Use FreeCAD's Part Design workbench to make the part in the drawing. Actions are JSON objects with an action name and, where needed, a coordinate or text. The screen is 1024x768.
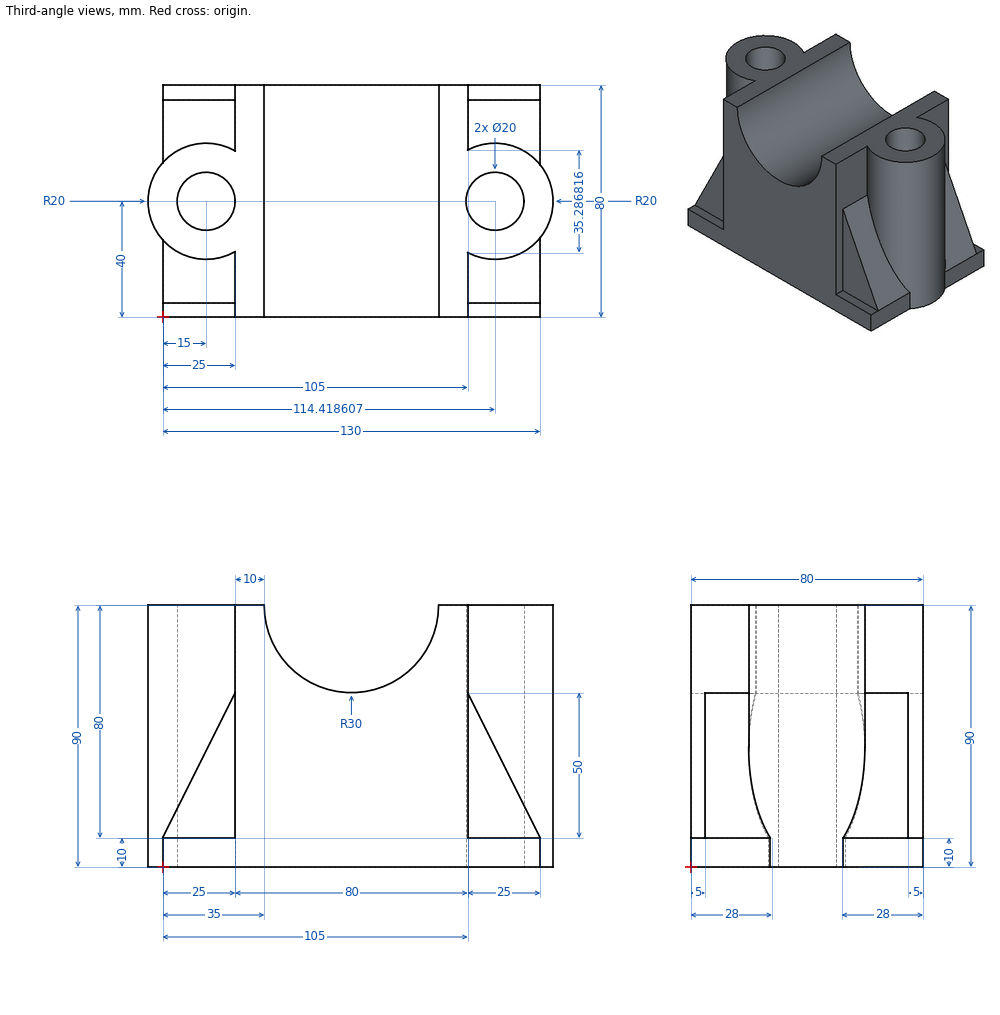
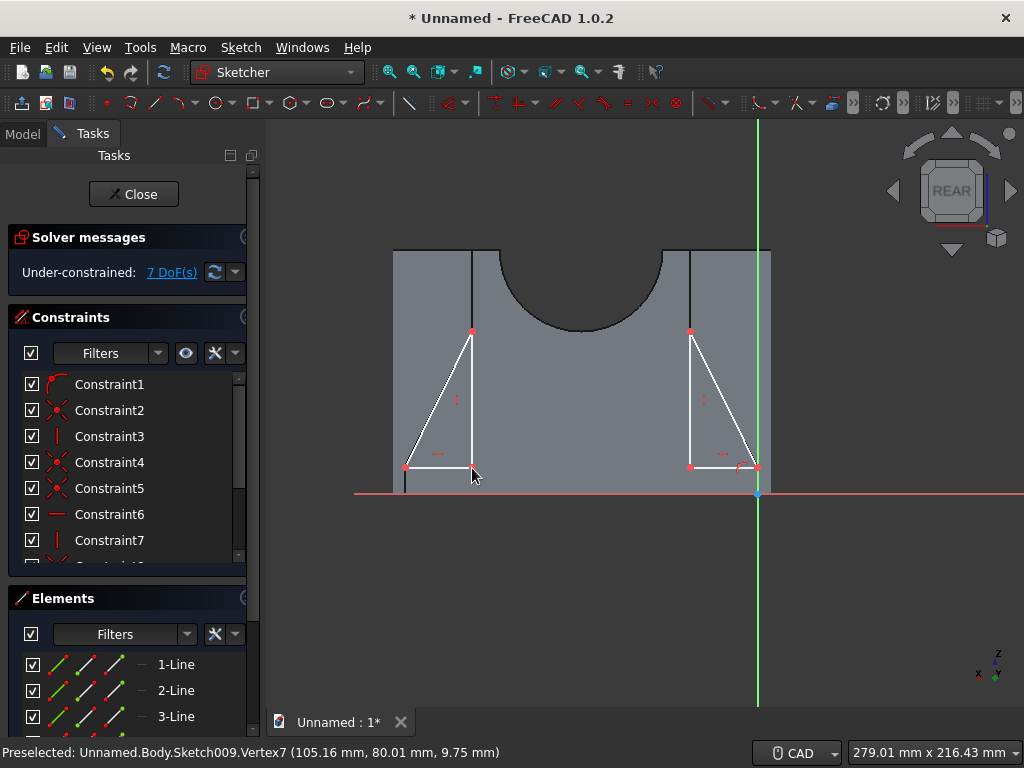
{"action": "left_click", "coordinate": [448, 104]}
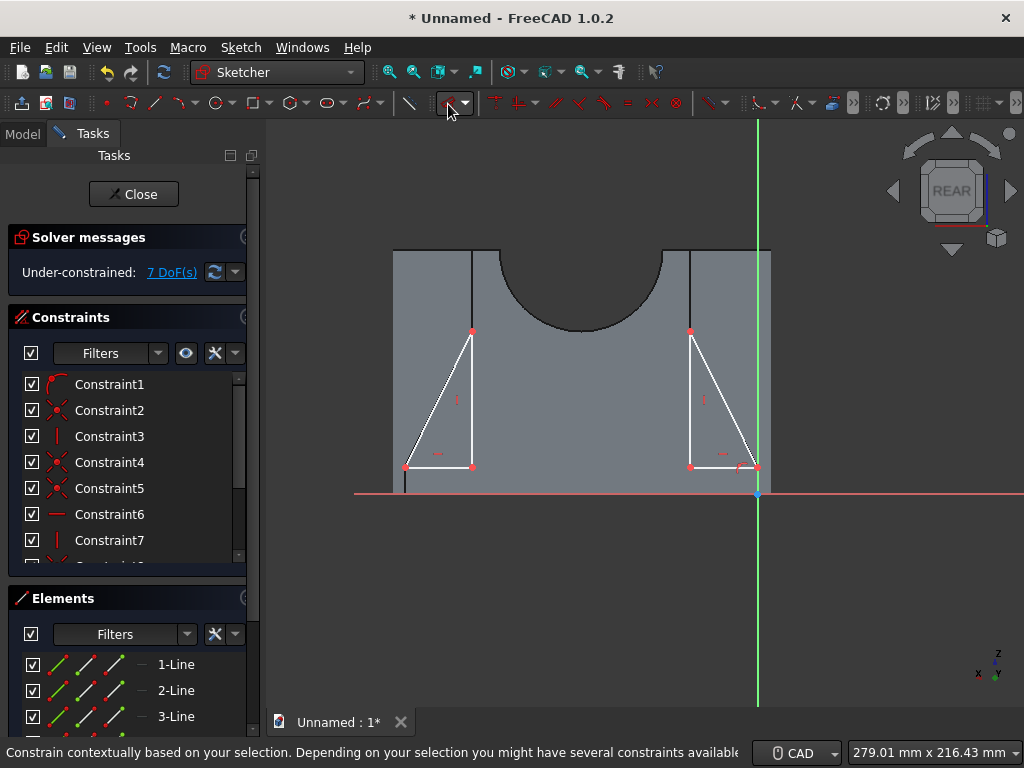
{"action": "left_click", "coordinate": [690, 373]}
{"action": "left_click", "coordinate": [724, 369]}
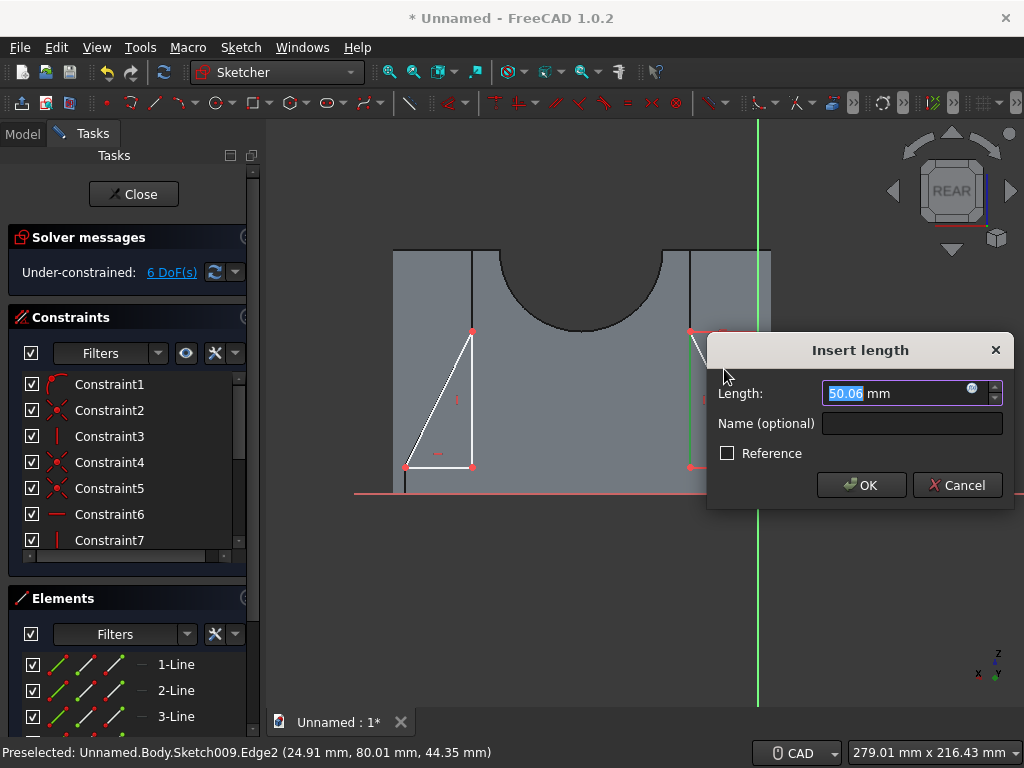
{"action": "type", "text": "50"}
{"action": "key", "text": "Return"}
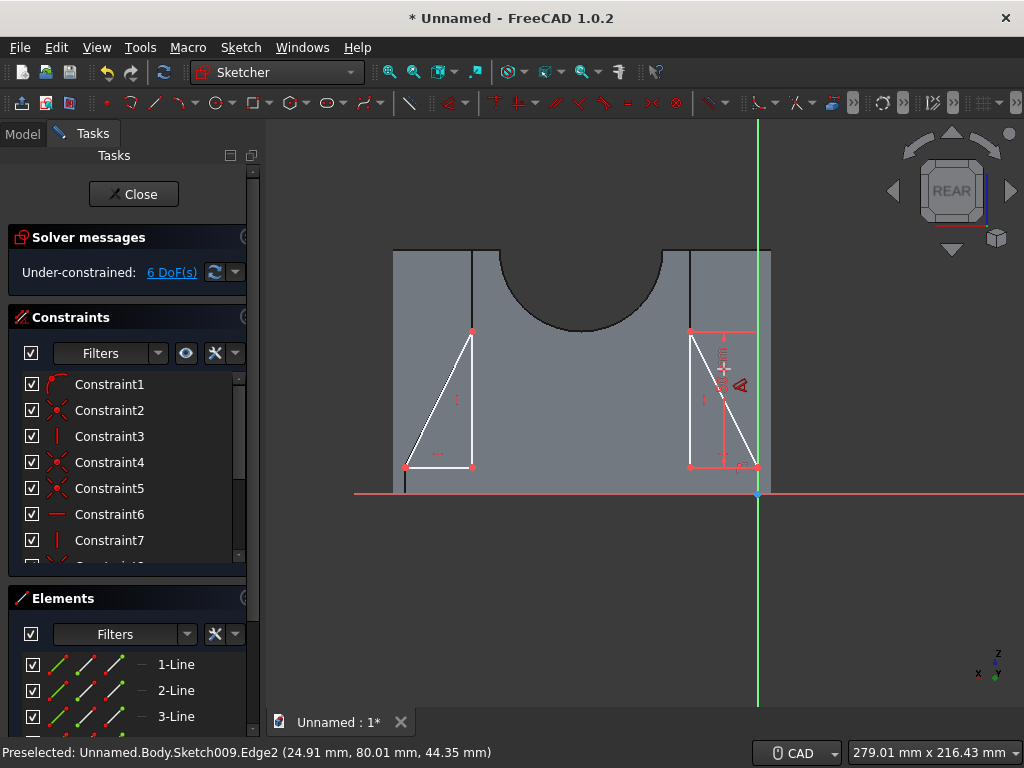
{"action": "left_click", "coordinate": [710, 468]}
{"action": "left_click", "coordinate": [724, 434]}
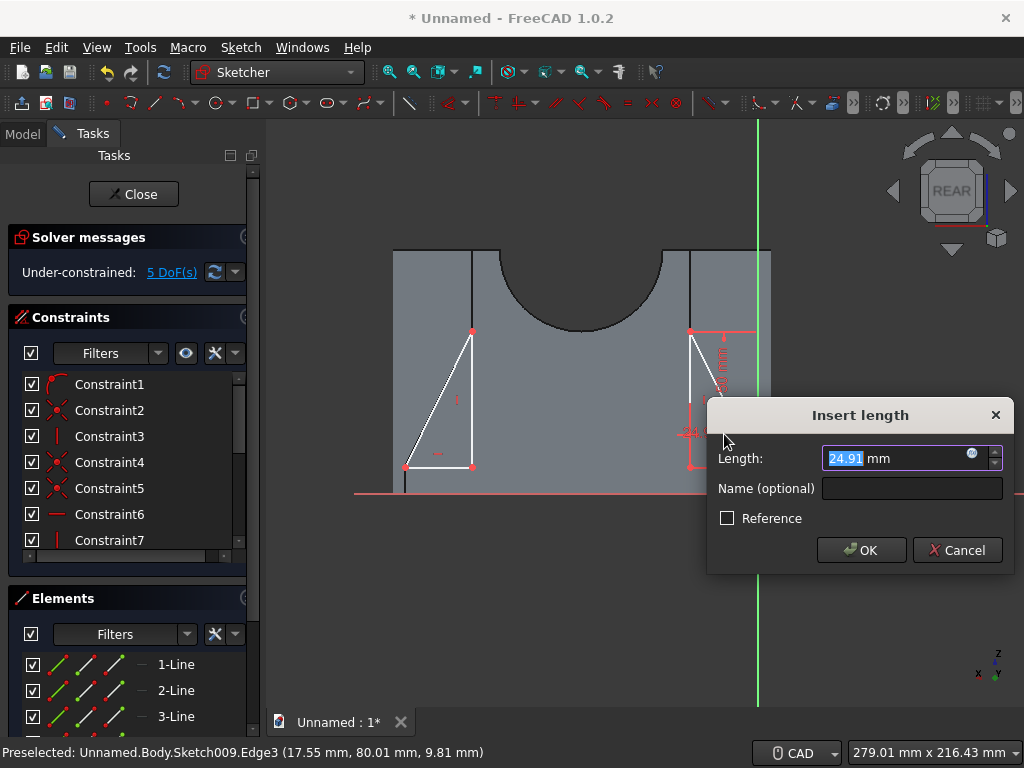
{"action": "type", "text": "25"}
{"action": "key", "text": "Return"}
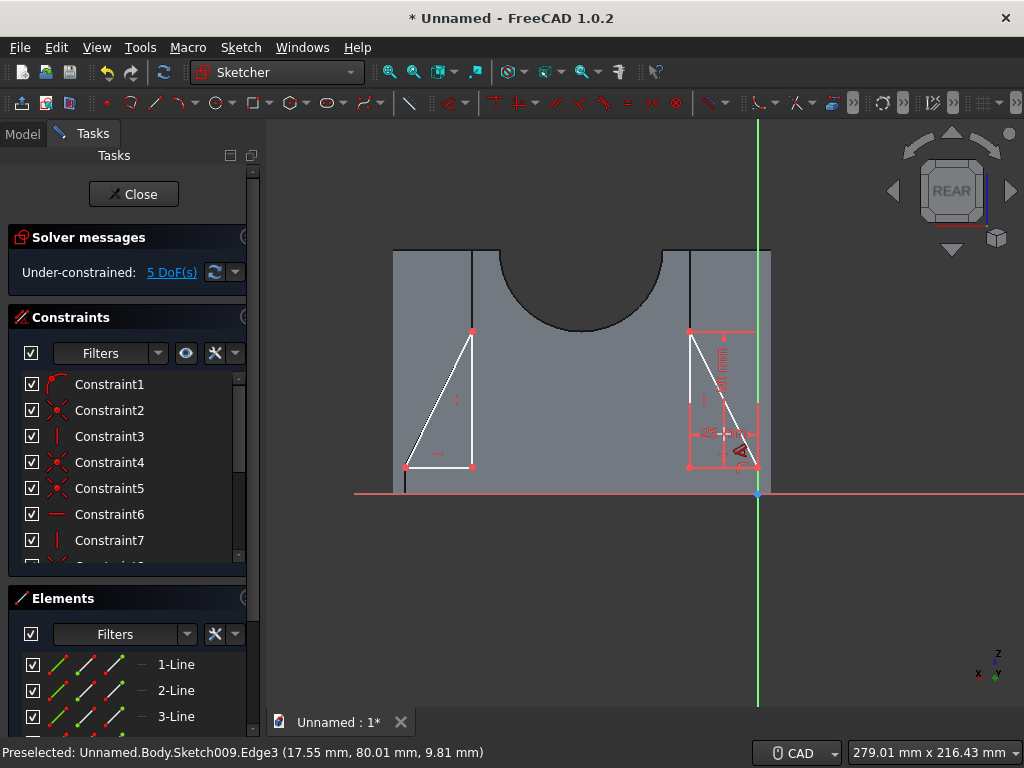
{"action": "left_click", "coordinate": [472, 427]}
{"action": "left_click", "coordinate": [438, 369]}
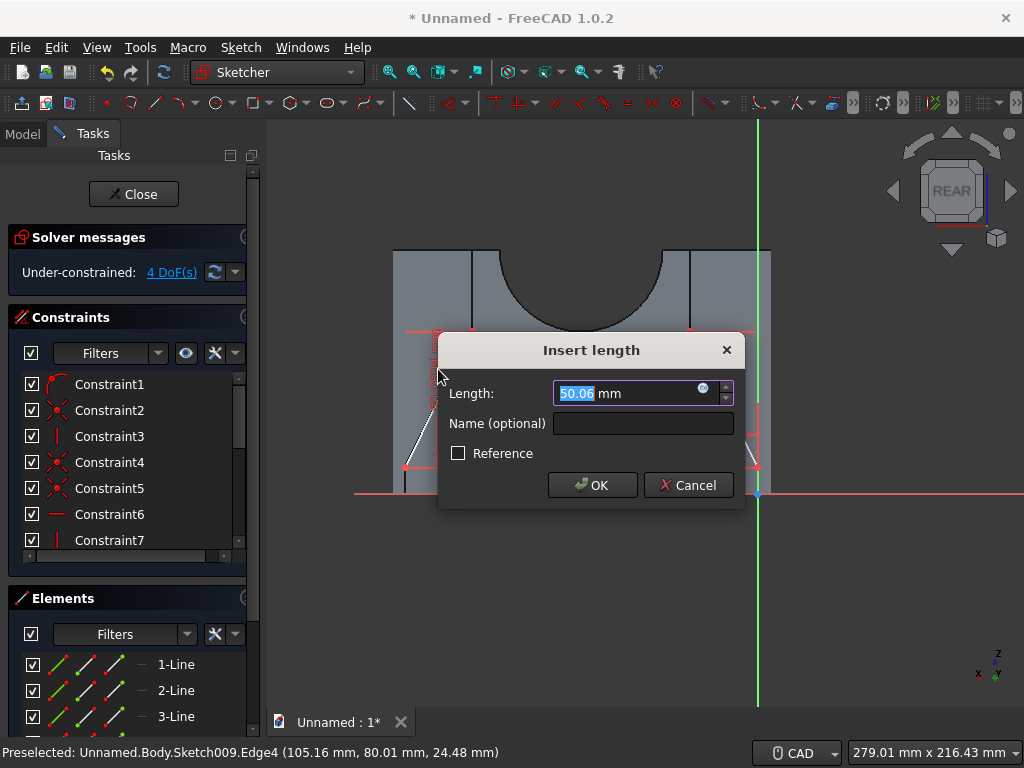
{"action": "type", "text": "50"}
{"action": "key", "text": "Return"}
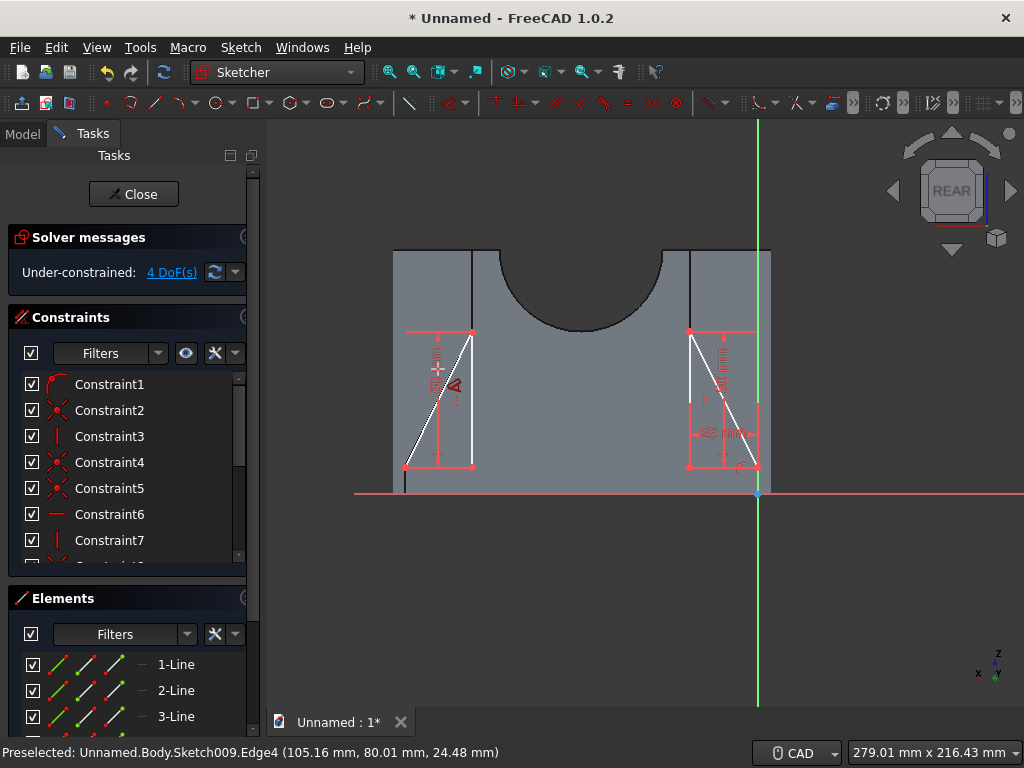
{"action": "left_click", "coordinate": [425, 468]}
{"action": "left_click", "coordinate": [439, 434]}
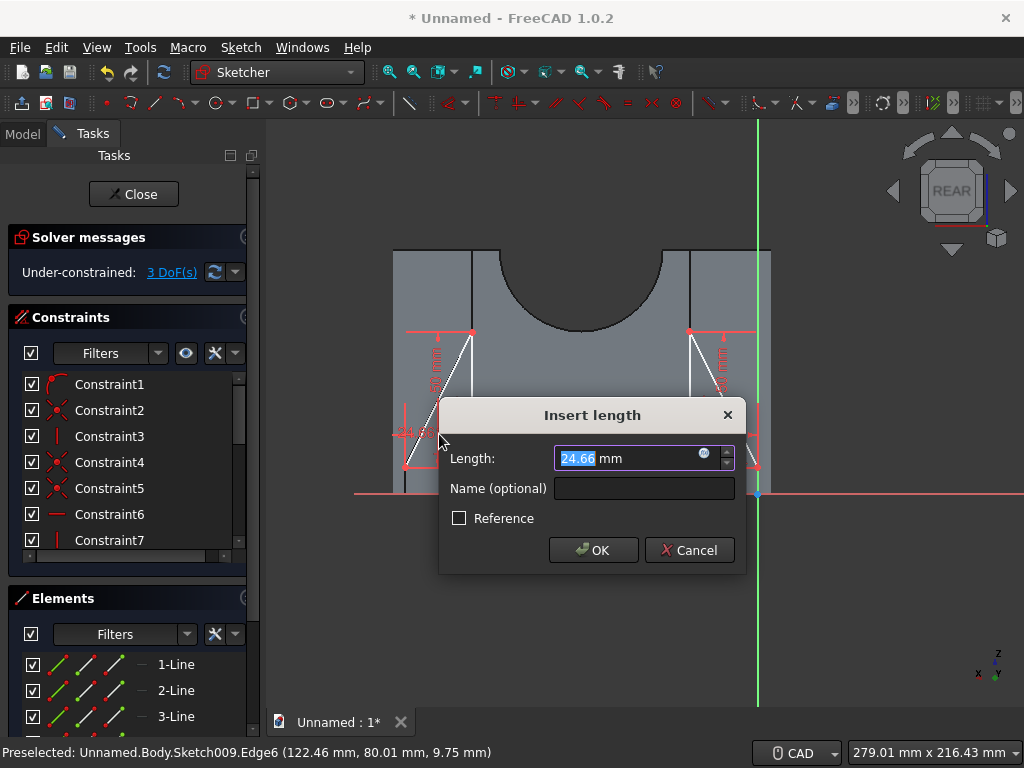
{"action": "type", "text": "25"}
{"action": "key", "text": "Return"}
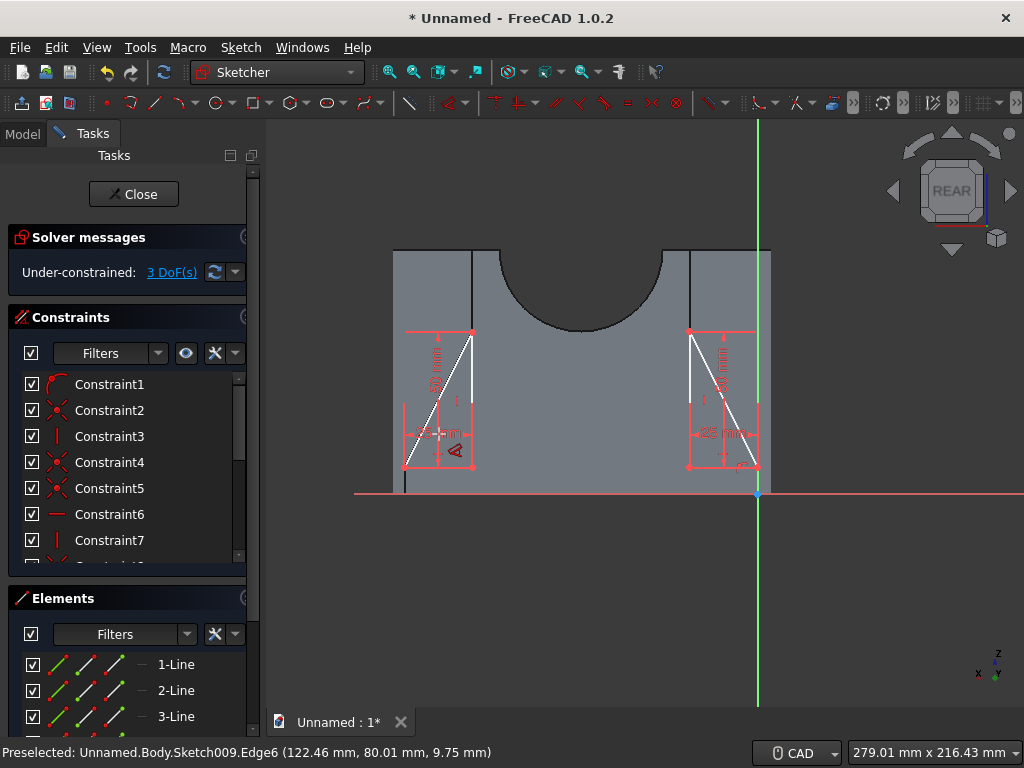
{"action": "scroll", "coordinate": [758, 468], "scroll_direction": "up", "scroll_amount": 2}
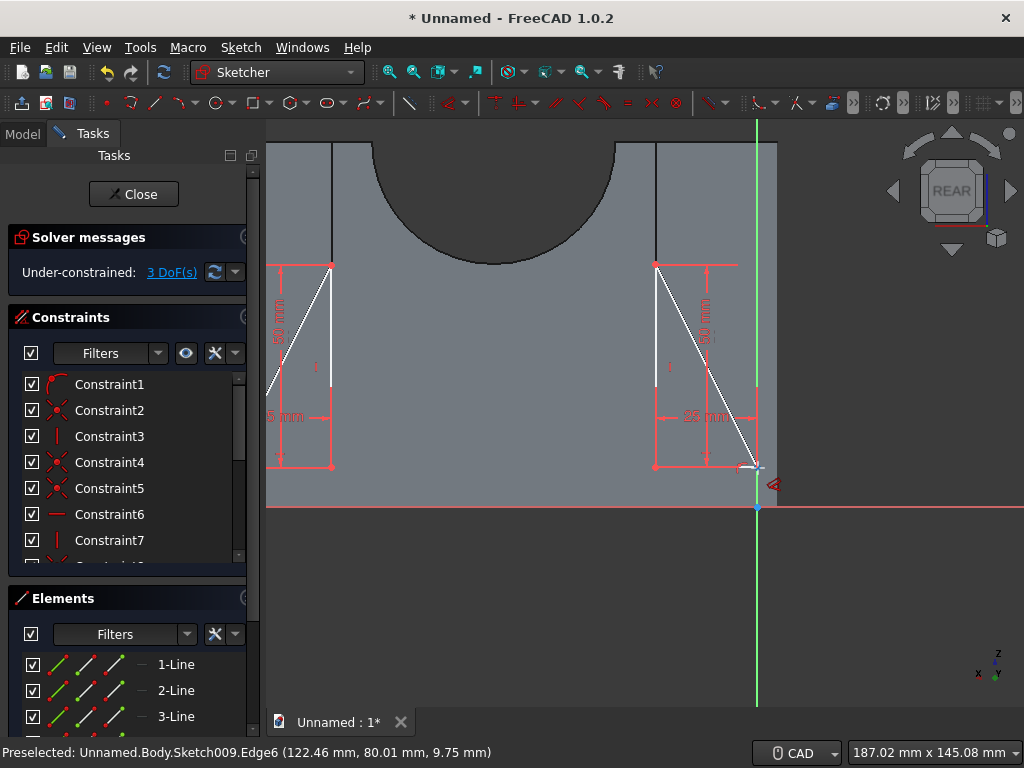
{"action": "left_click", "coordinate": [757, 467]}
{"action": "left_click", "coordinate": [791, 487]}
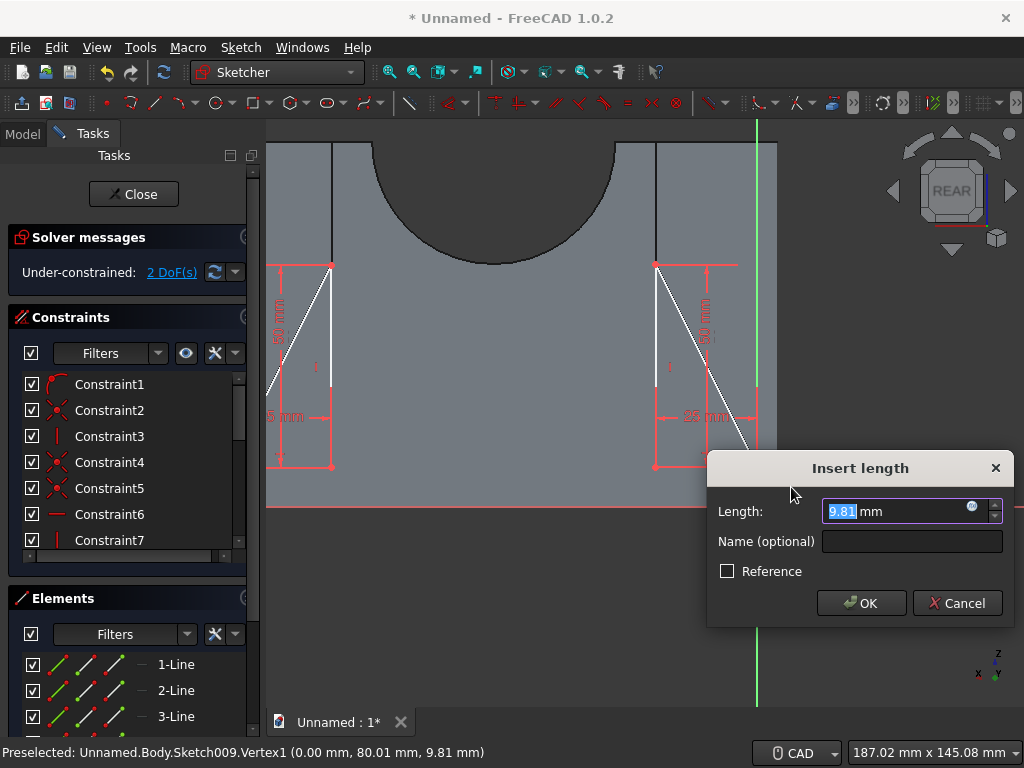
{"action": "type", "text": "10"}
{"action": "key", "text": "Return"}